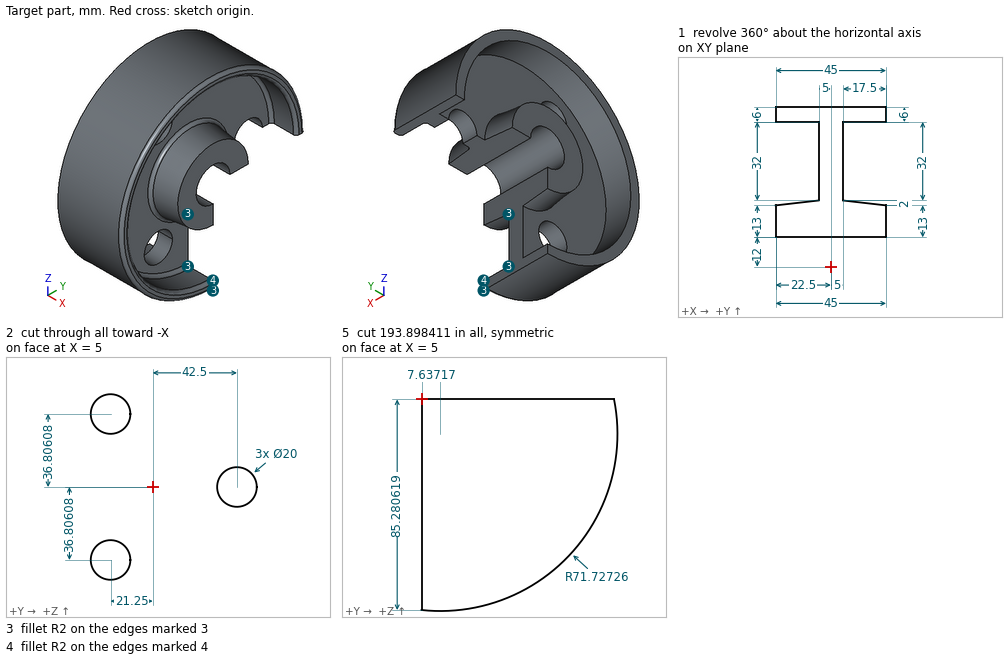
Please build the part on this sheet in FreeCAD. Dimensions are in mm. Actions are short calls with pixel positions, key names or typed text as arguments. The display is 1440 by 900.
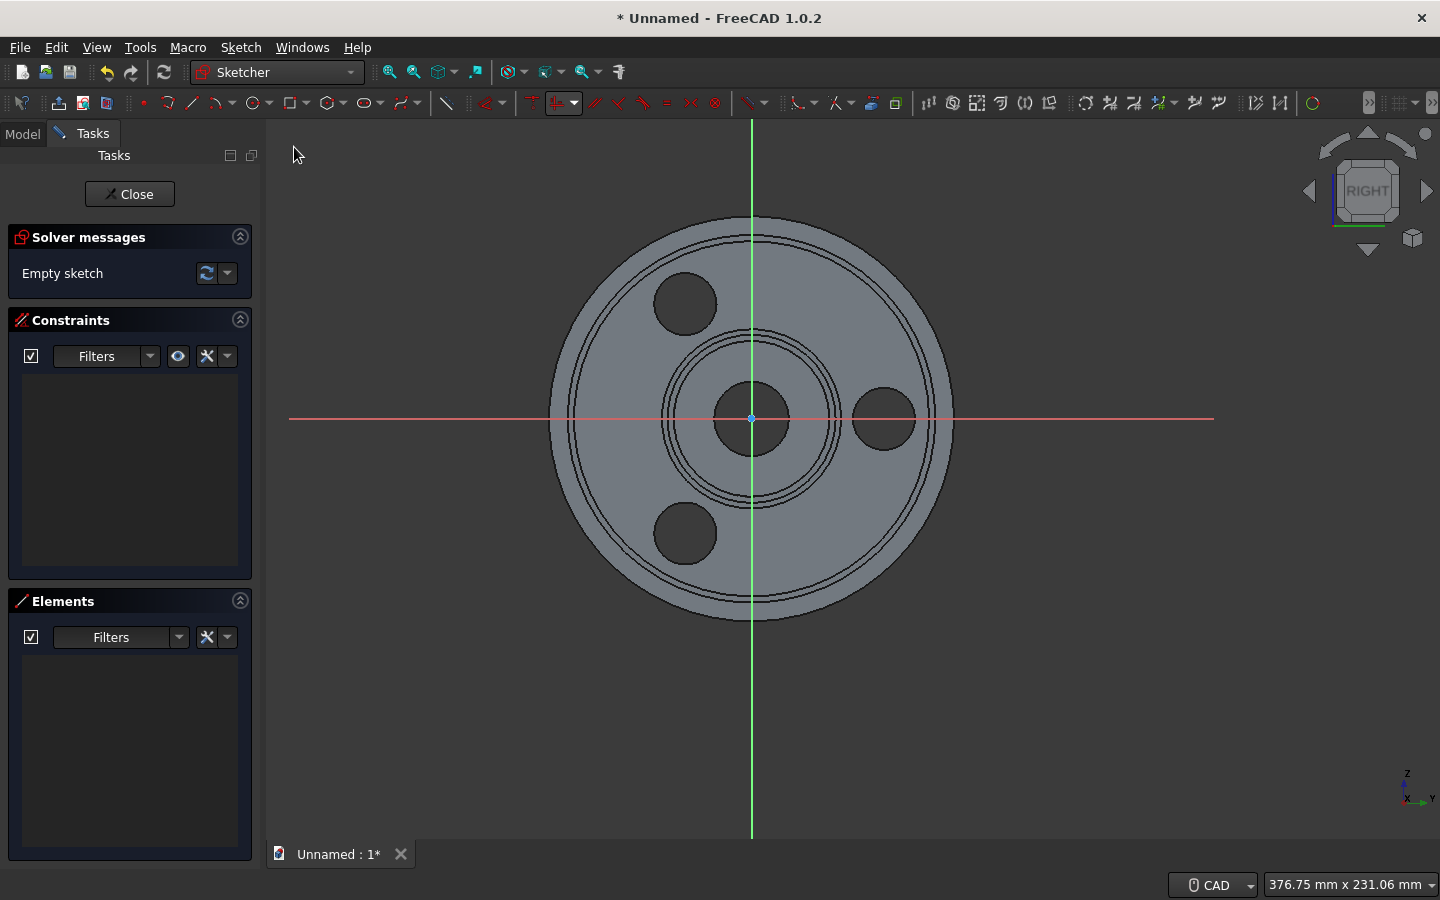
scroll(981, 640, up, 3)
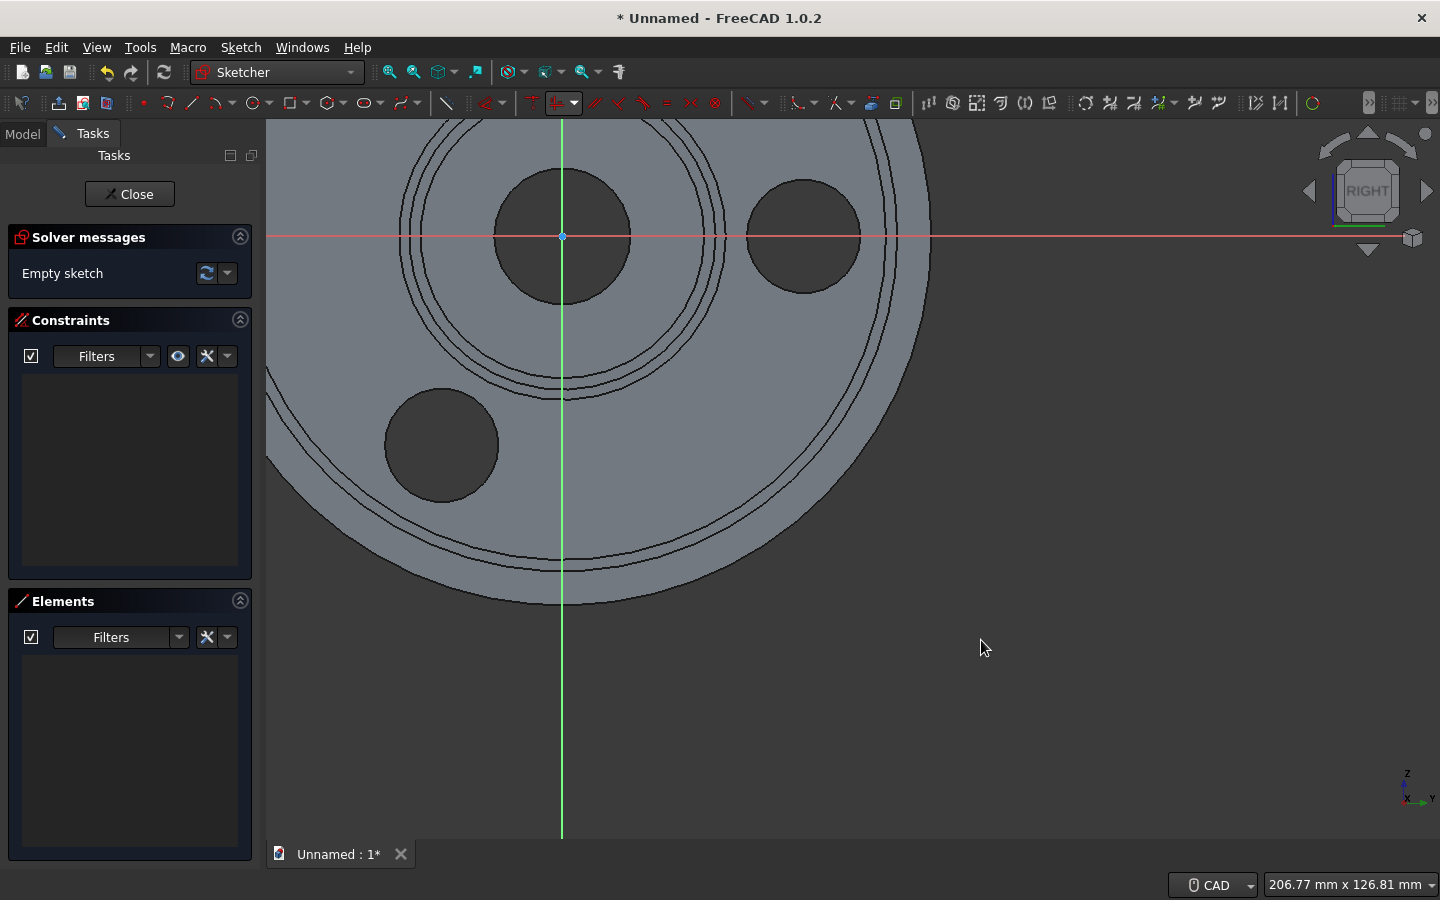
click(168, 104)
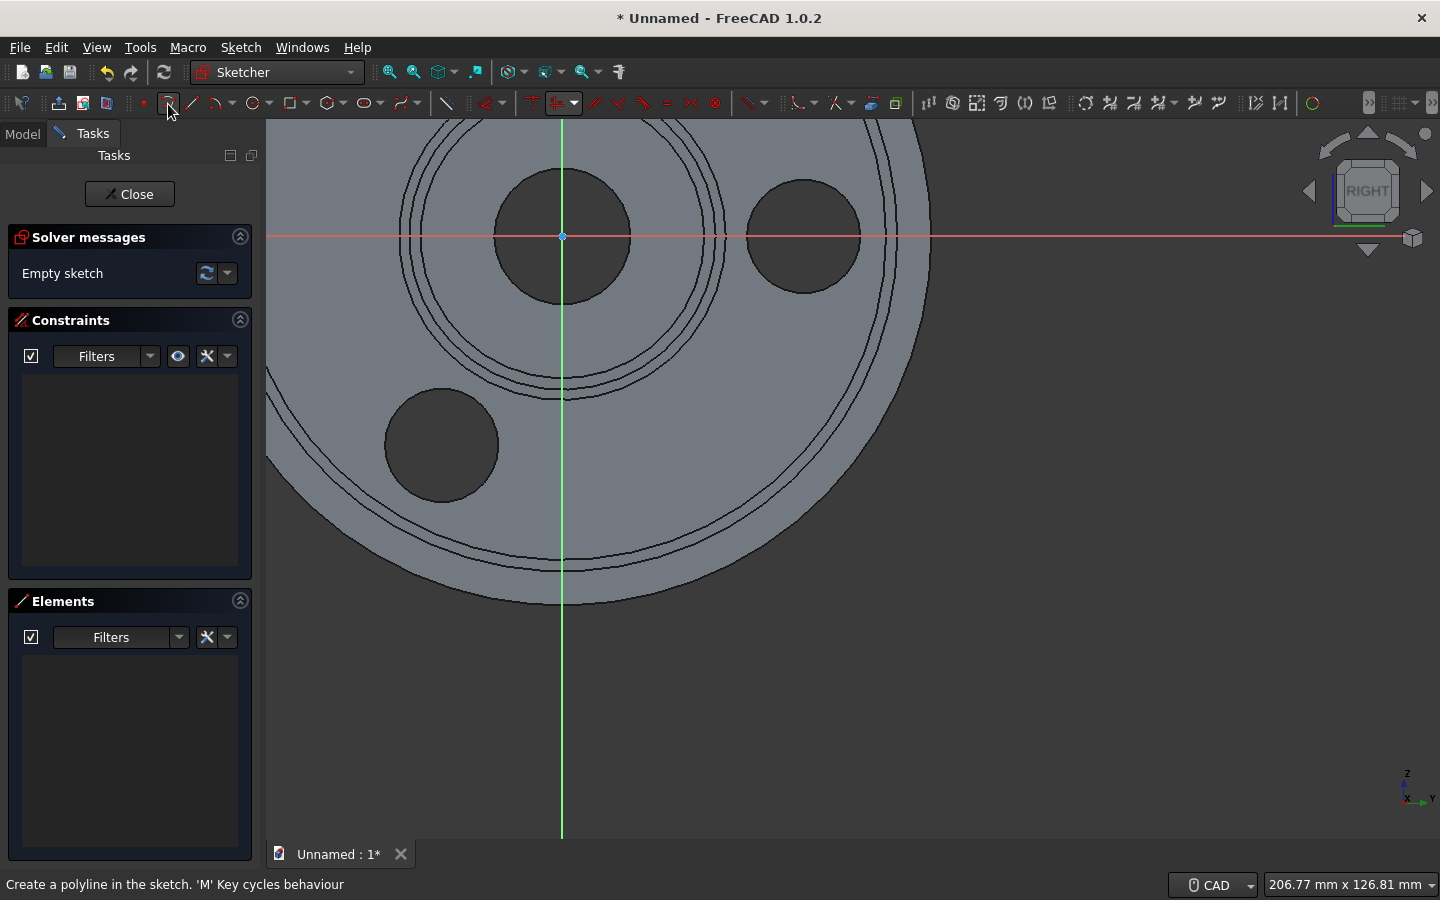
click(1005, 236)
click(562, 236)
click(571, 721)
right_click(571, 721)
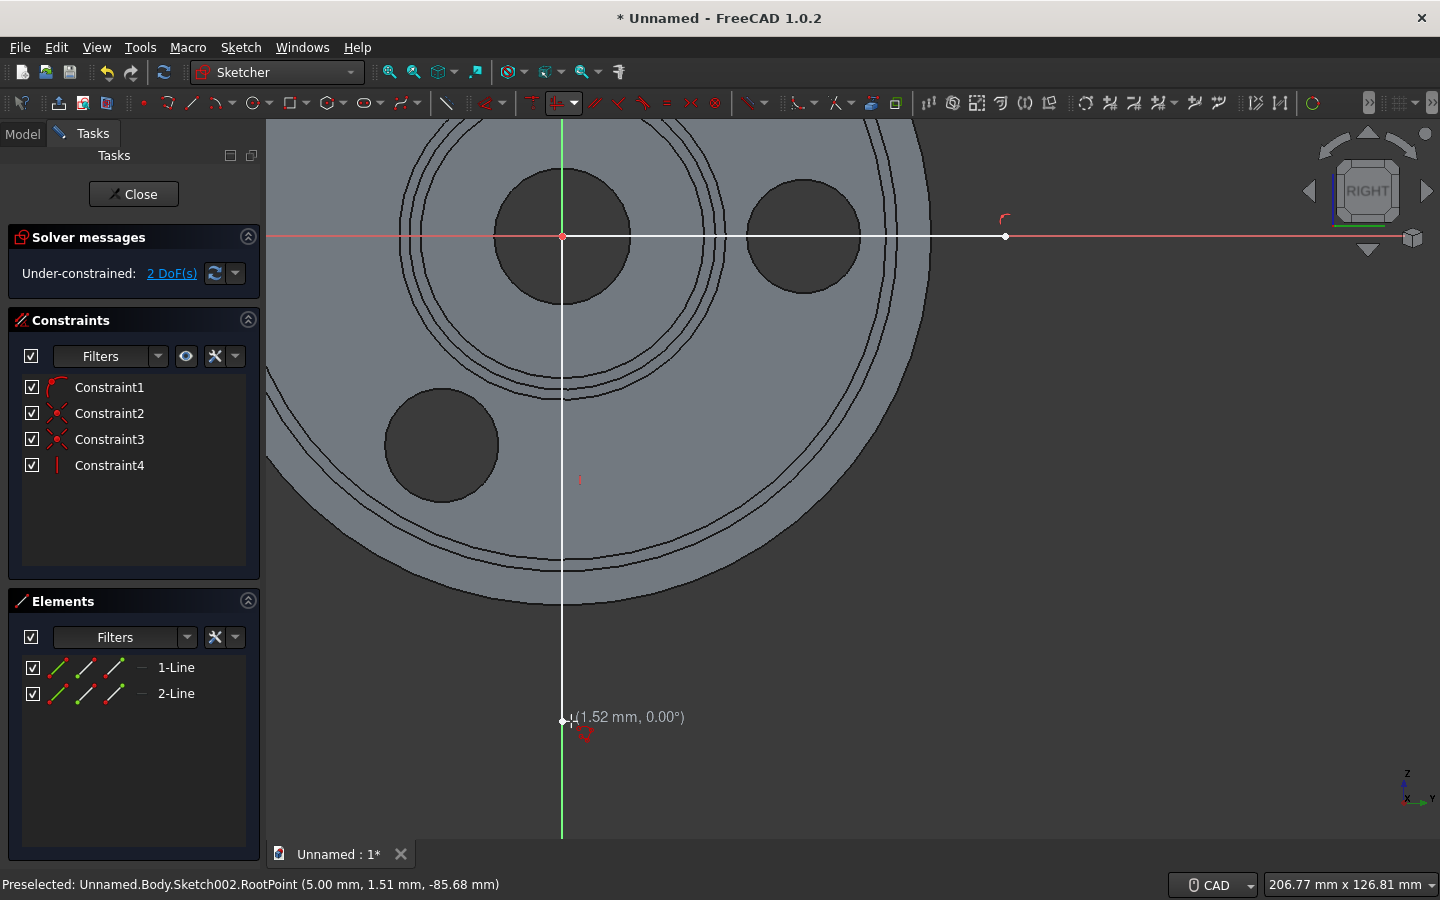
key(g)
key(3)
key(a)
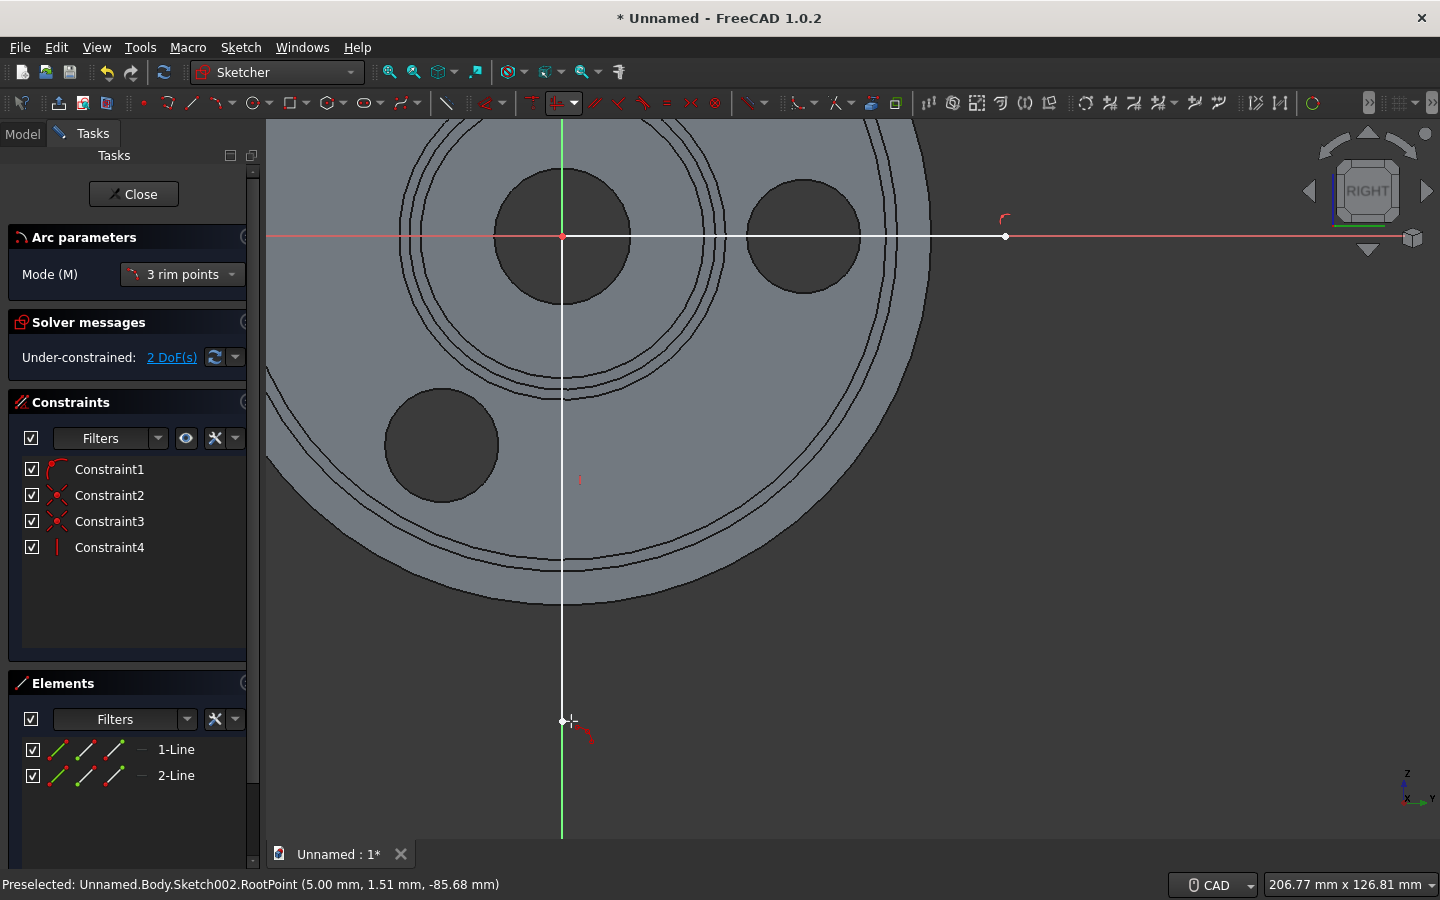
click(562, 722)
click(1005, 236)
click(906, 591)
key(Escape)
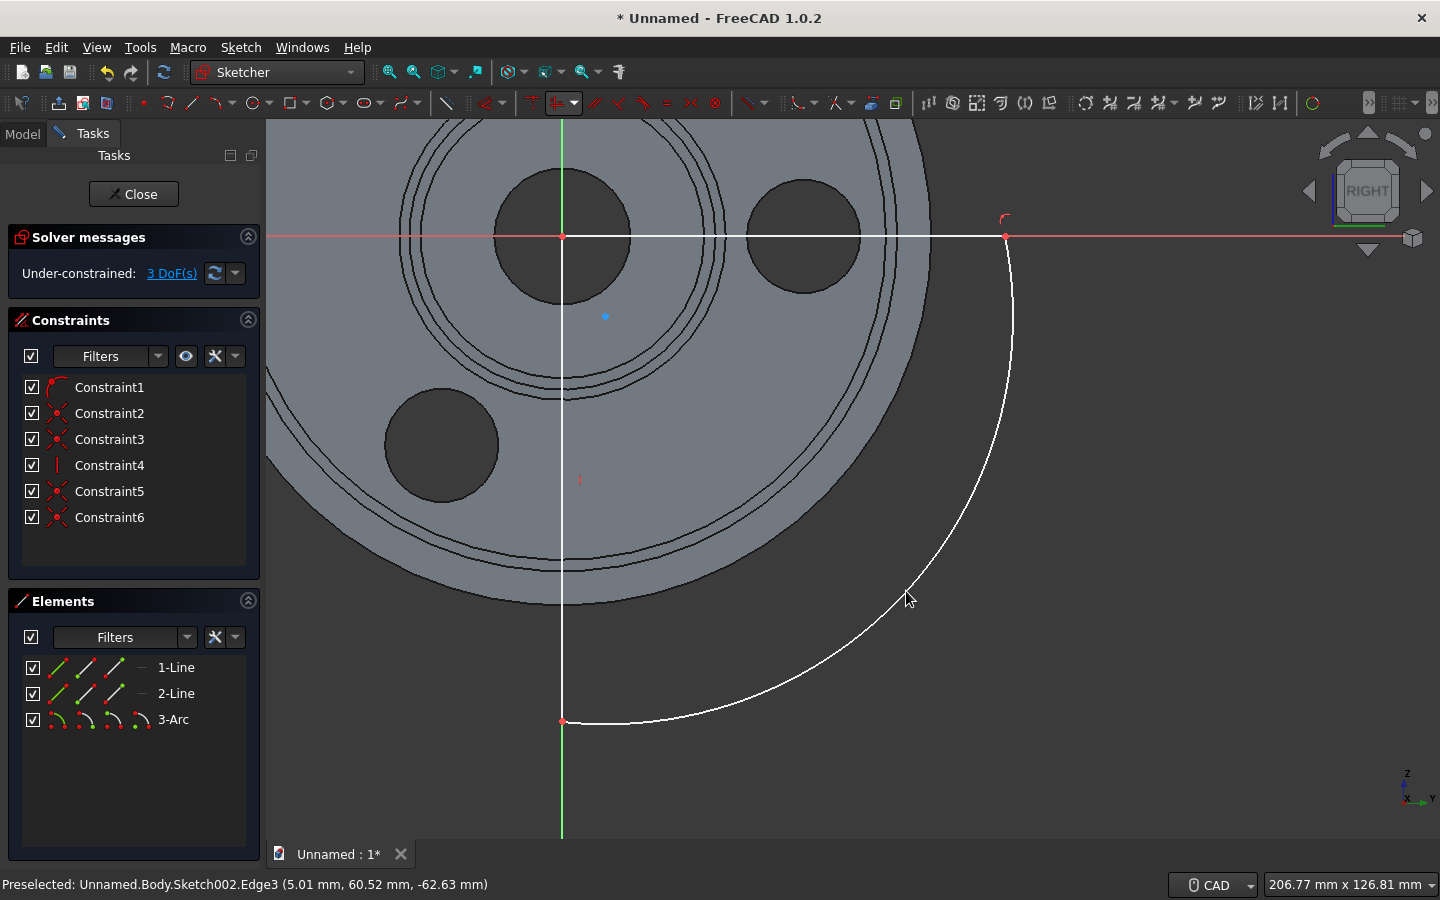
click(486, 104)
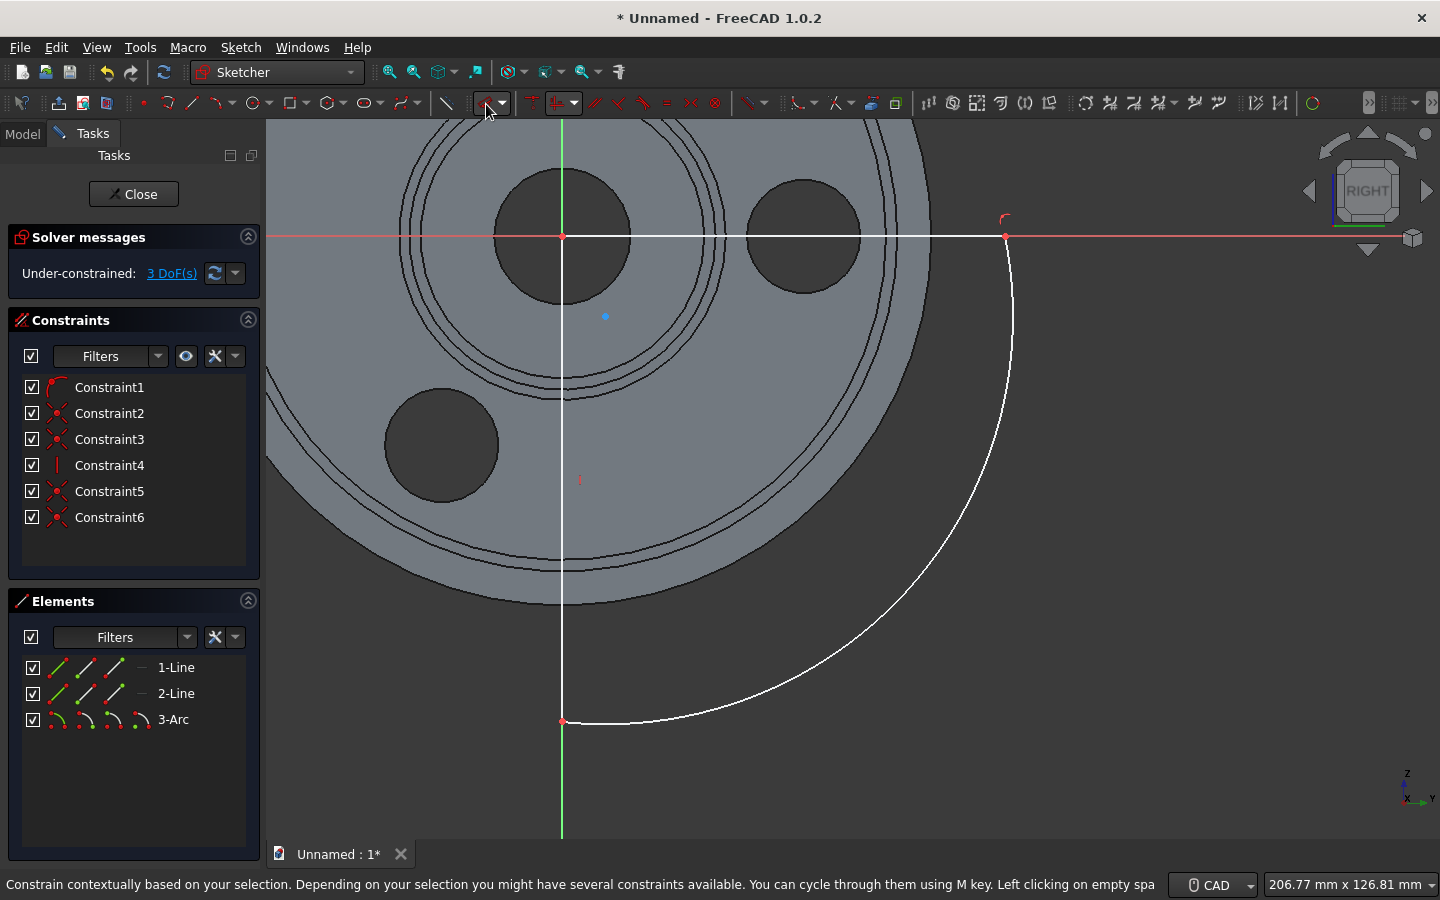
click(785, 683)
click(799, 712)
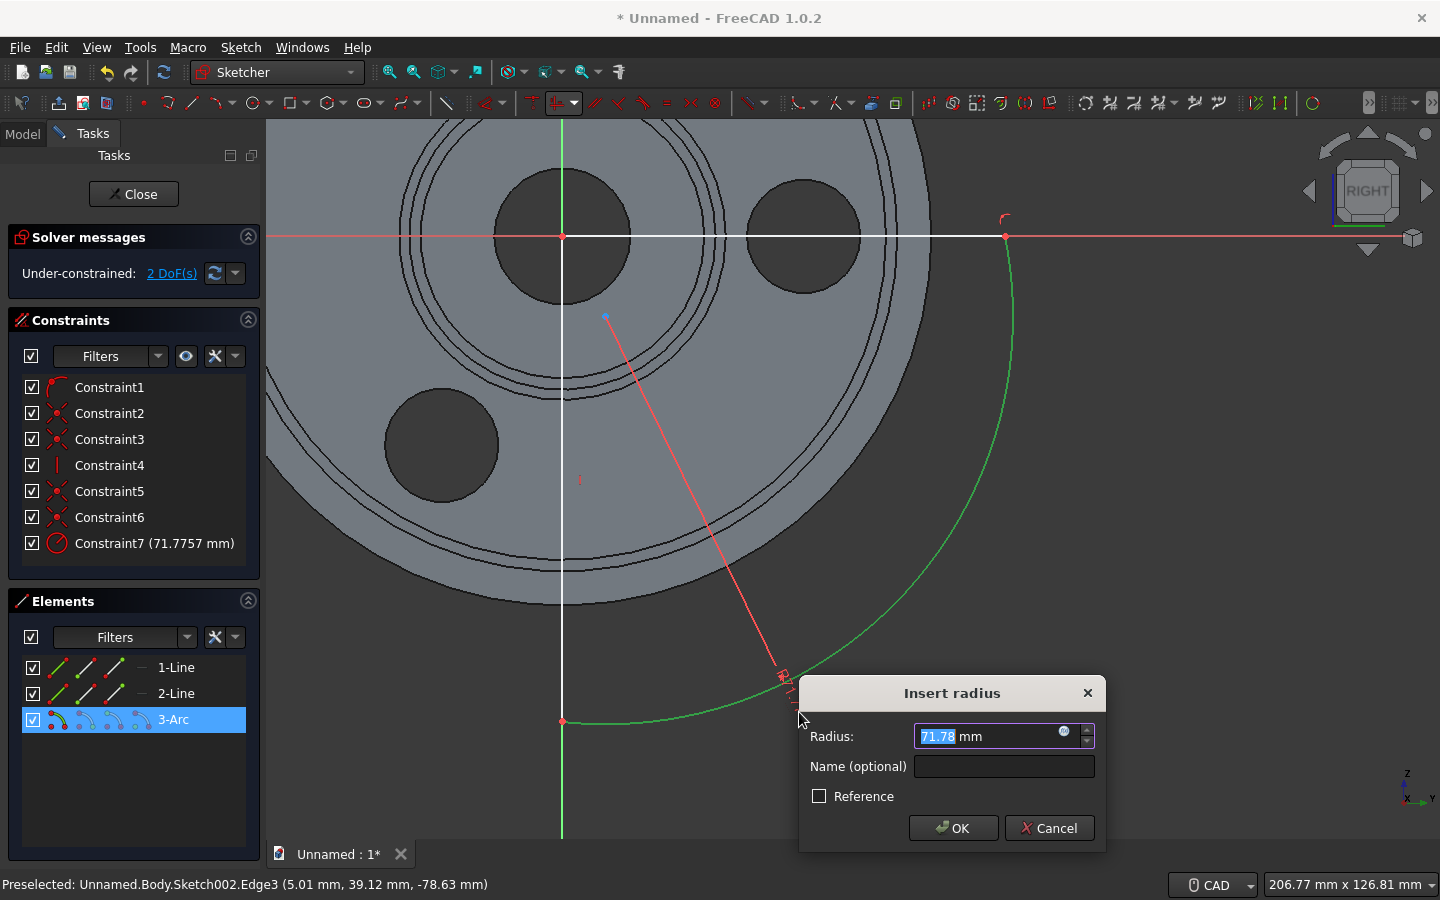
text(71.72726)
key(Return)